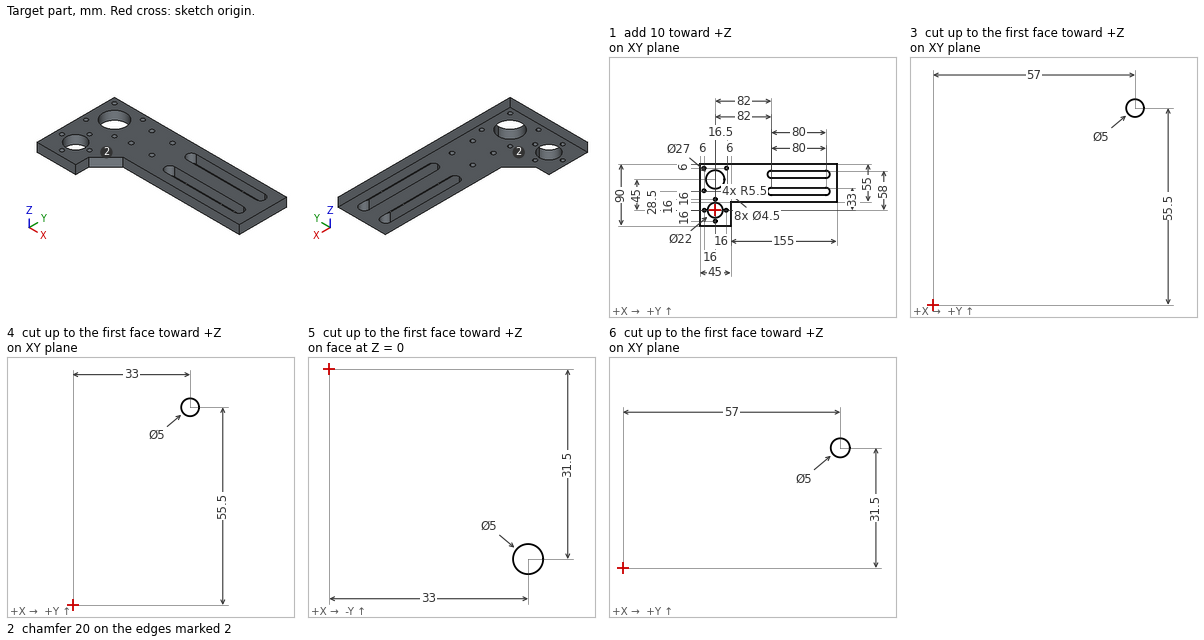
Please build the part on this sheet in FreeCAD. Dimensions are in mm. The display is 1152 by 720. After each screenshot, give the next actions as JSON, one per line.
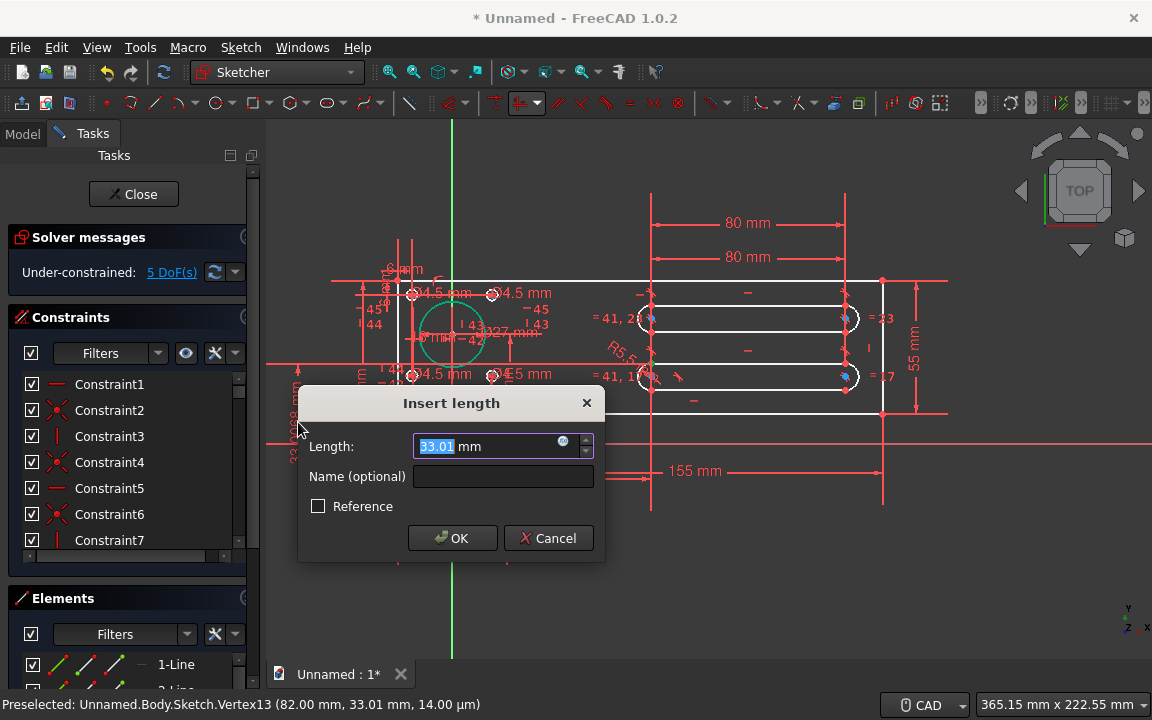
{"action": "type", "text": "33"}
{"action": "key", "text": "Return"}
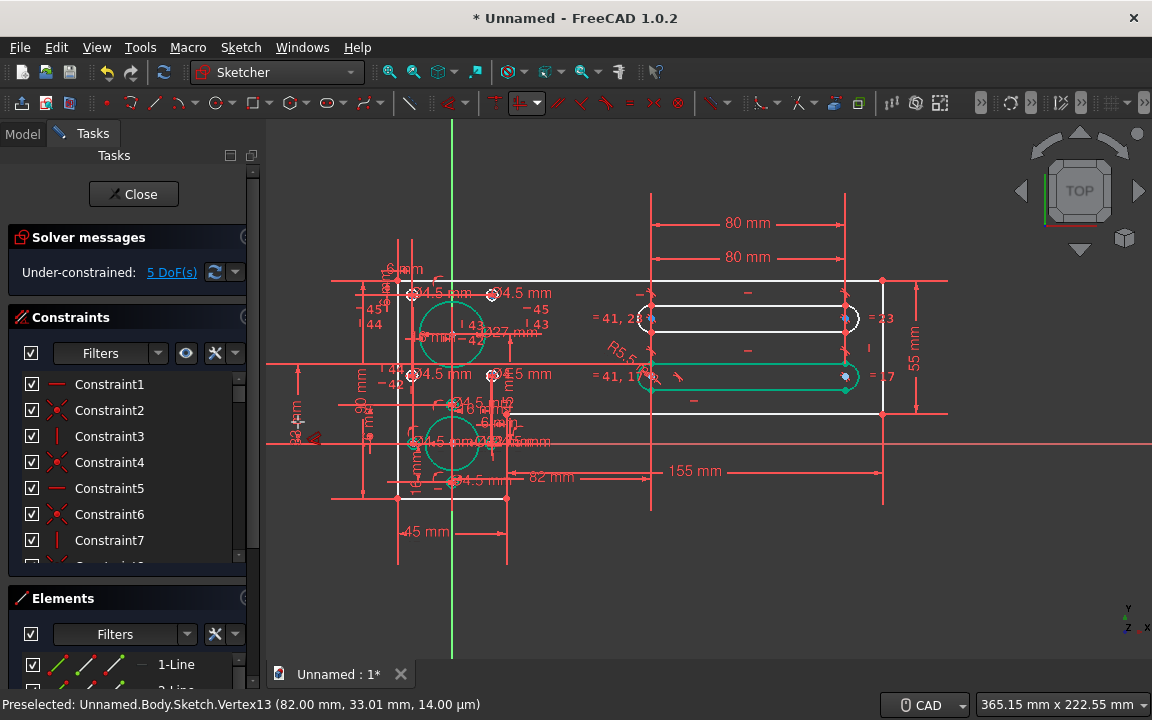
{"action": "left_click", "coordinate": [651, 306]}
{"action": "left_click", "coordinate": [552, 248]}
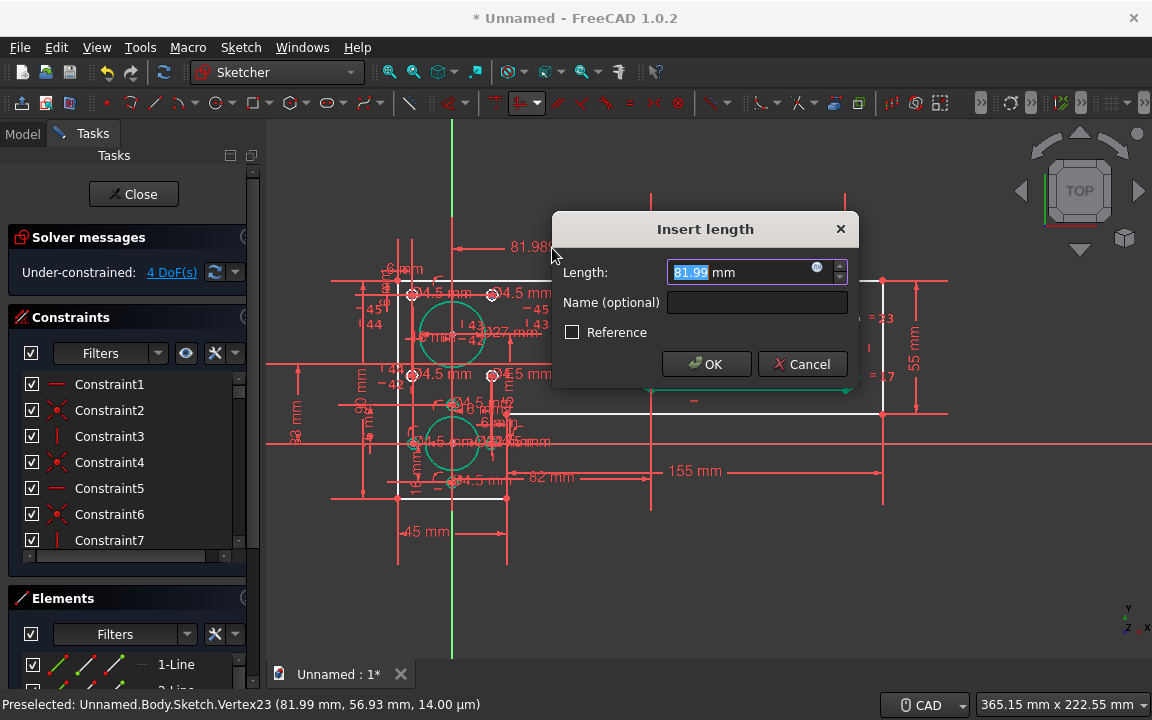
{"action": "type", "text": "82"}
{"action": "key", "text": "Return"}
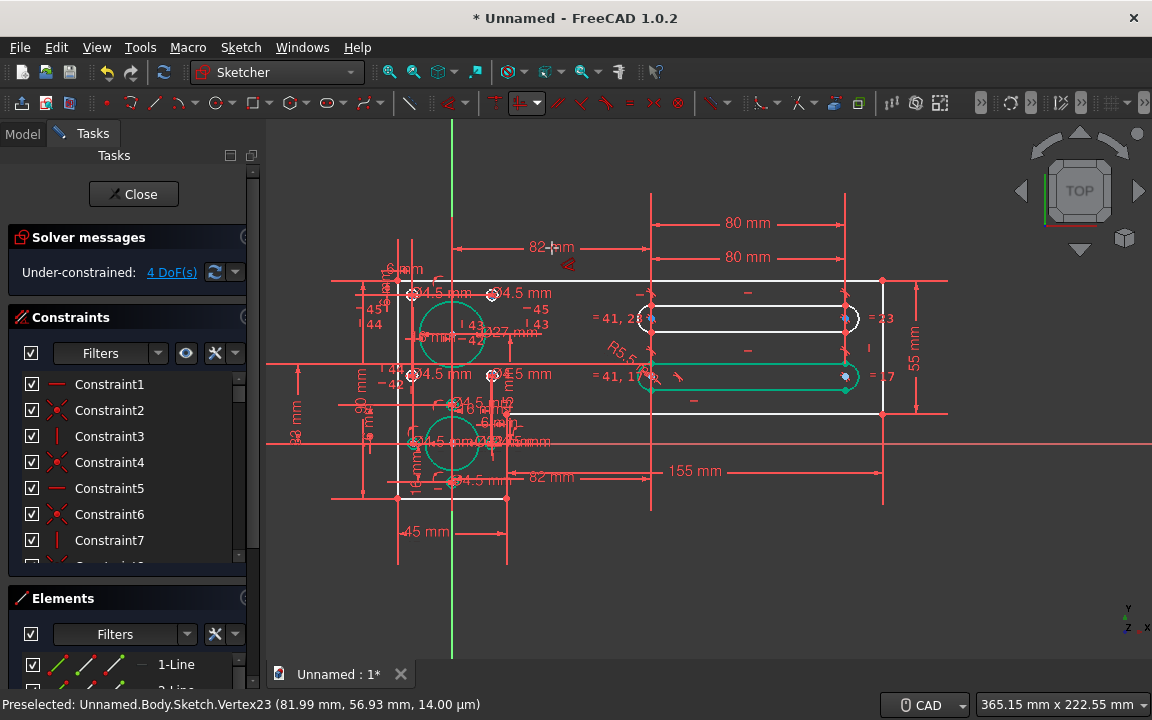
{"action": "left_click", "coordinate": [651, 306]}
{"action": "left_click", "coordinate": [346, 343]}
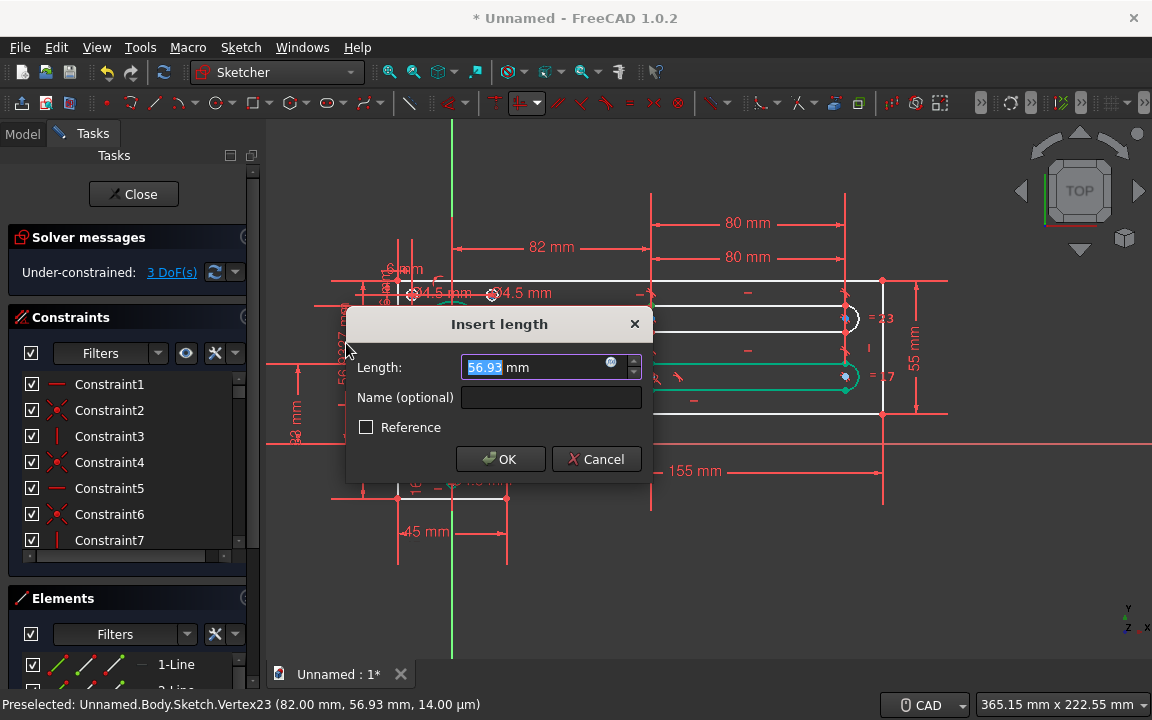
{"action": "type", "text": "58"}
{"action": "key", "text": "Return"}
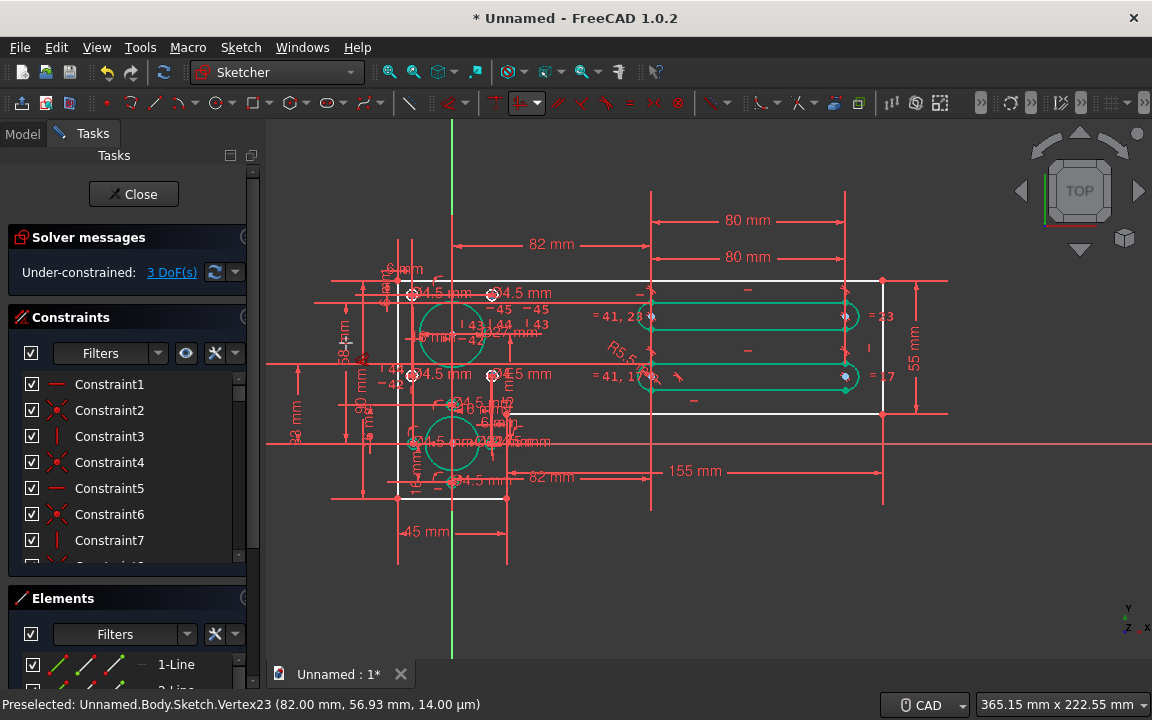
{"action": "left_click", "coordinate": [507, 414]}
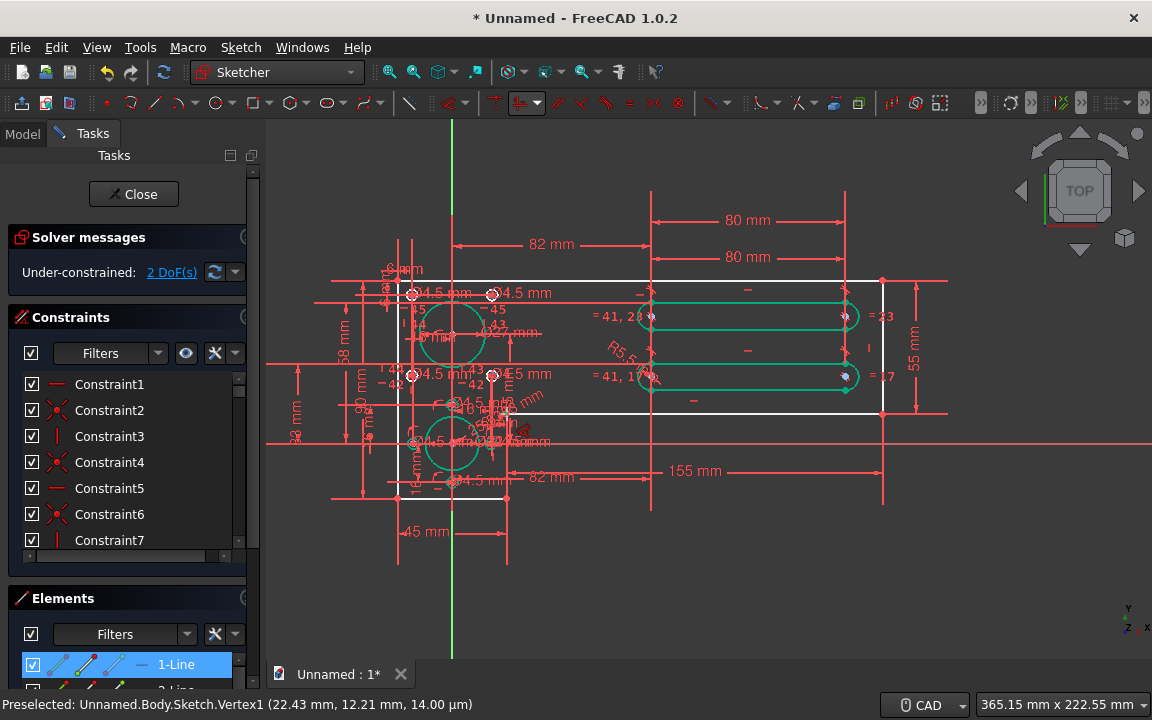
{"action": "left_click", "coordinate": [492, 376]}
{"action": "left_click", "coordinate": [434, 386]}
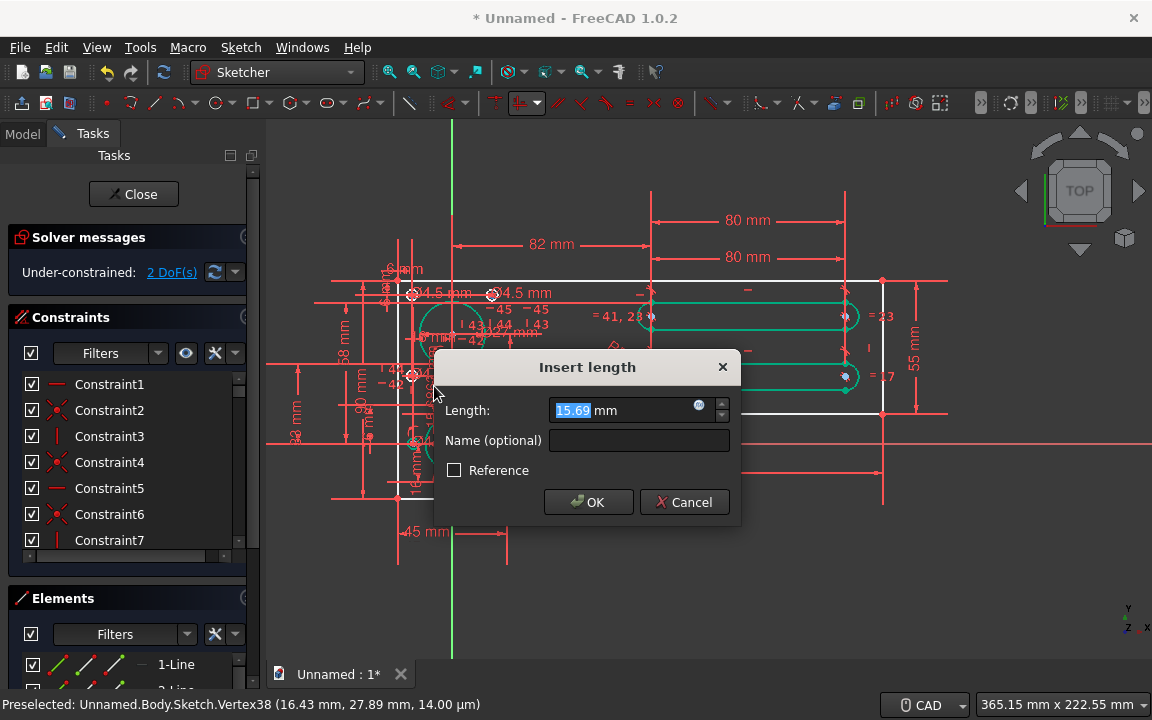
{"action": "type", "text": "16"}
{"action": "key", "text": "Return"}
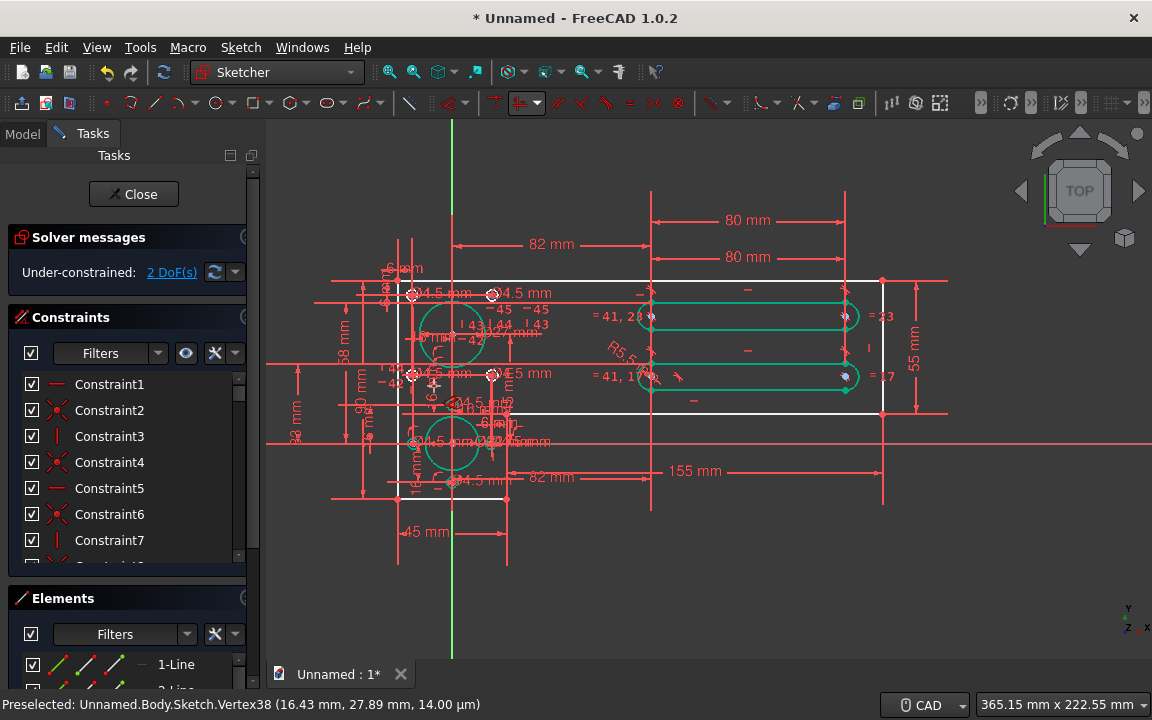
{"action": "left_click", "coordinate": [492, 375]}
{"action": "left_click", "coordinate": [472, 574]}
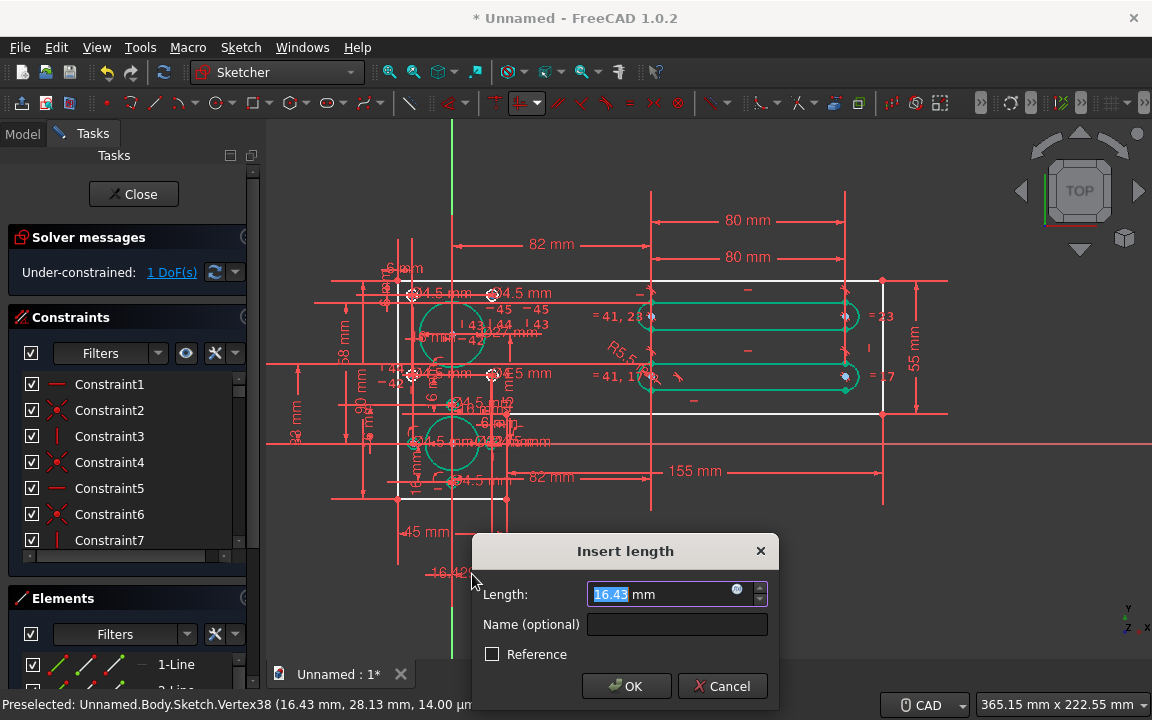
{"action": "type", "text": "16.5"}
{"action": "key", "text": "Return"}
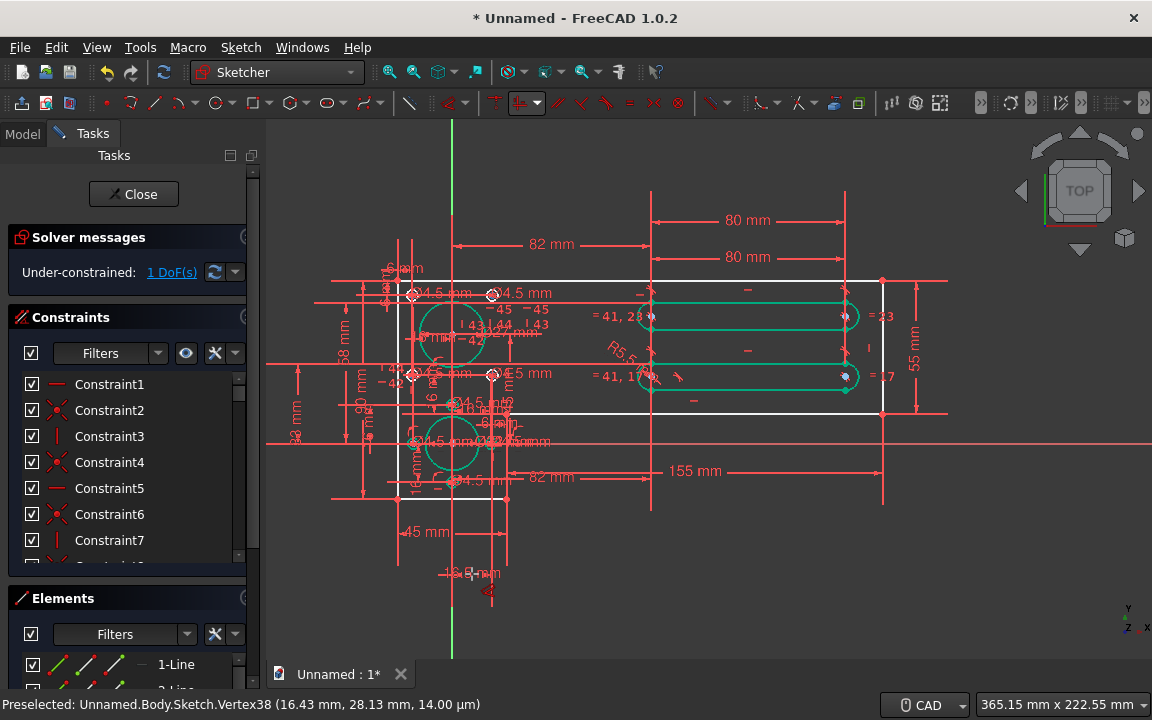
{"action": "left_click", "coordinate": [492, 375]}
{"action": "left_click", "coordinate": [598, 394]}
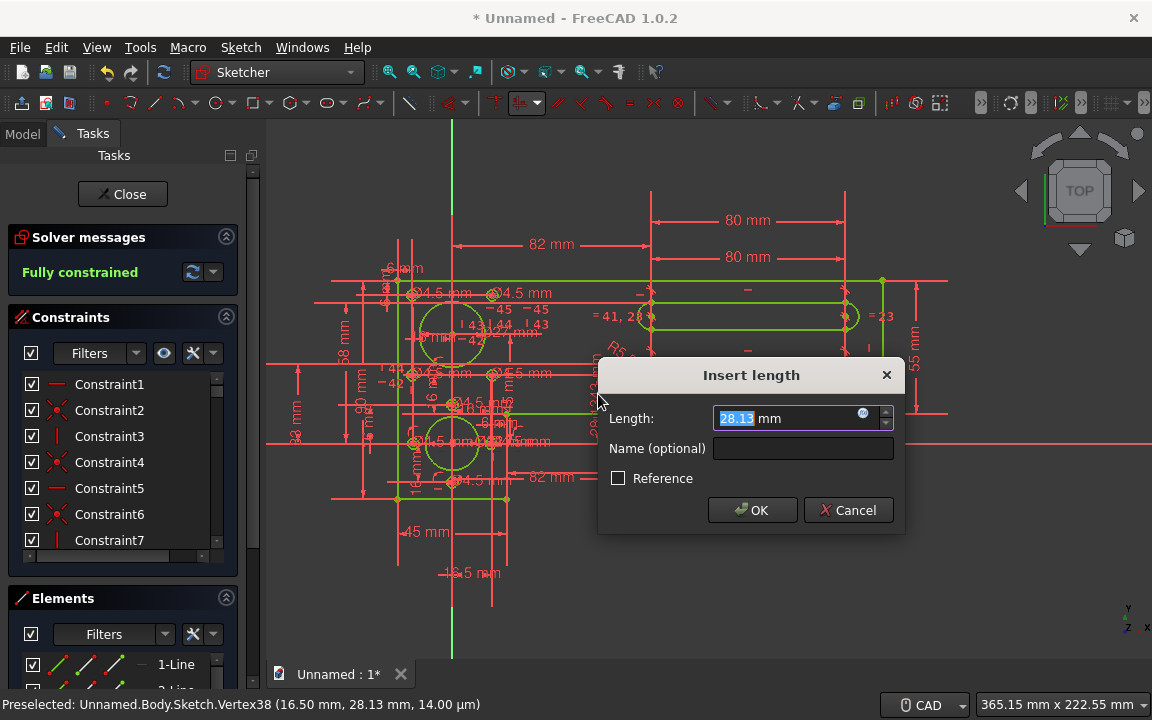
{"action": "type", "text": "28.5"}
{"action": "key", "text": "Return"}
{"action": "key", "text": "Escape"}